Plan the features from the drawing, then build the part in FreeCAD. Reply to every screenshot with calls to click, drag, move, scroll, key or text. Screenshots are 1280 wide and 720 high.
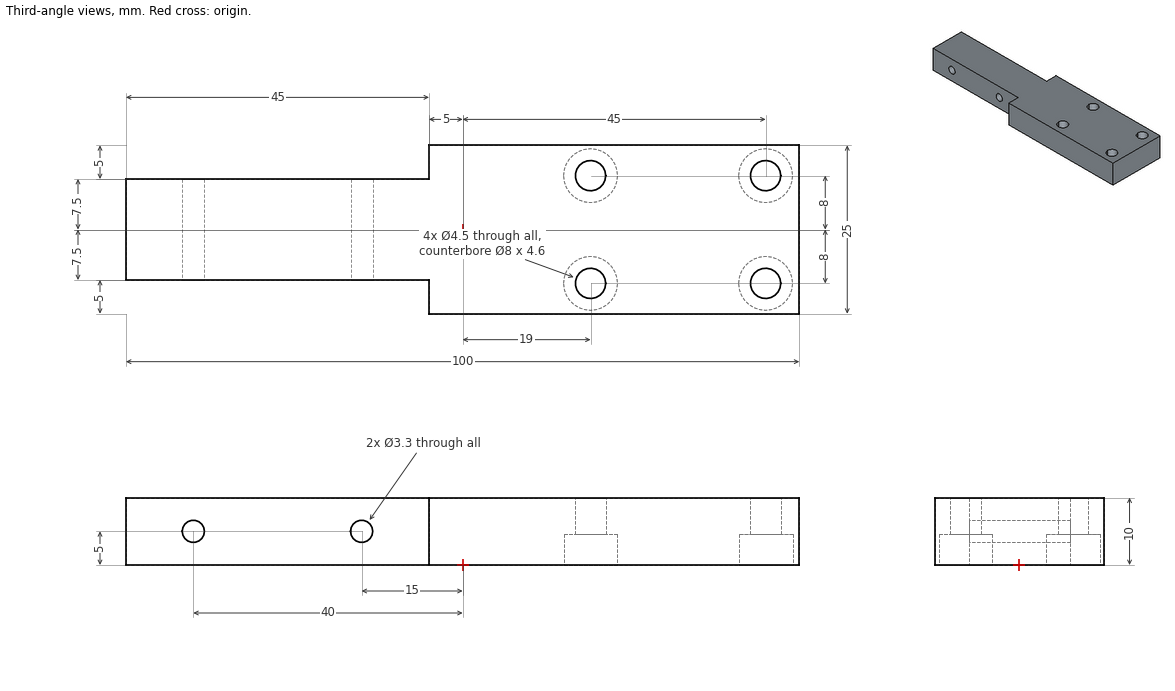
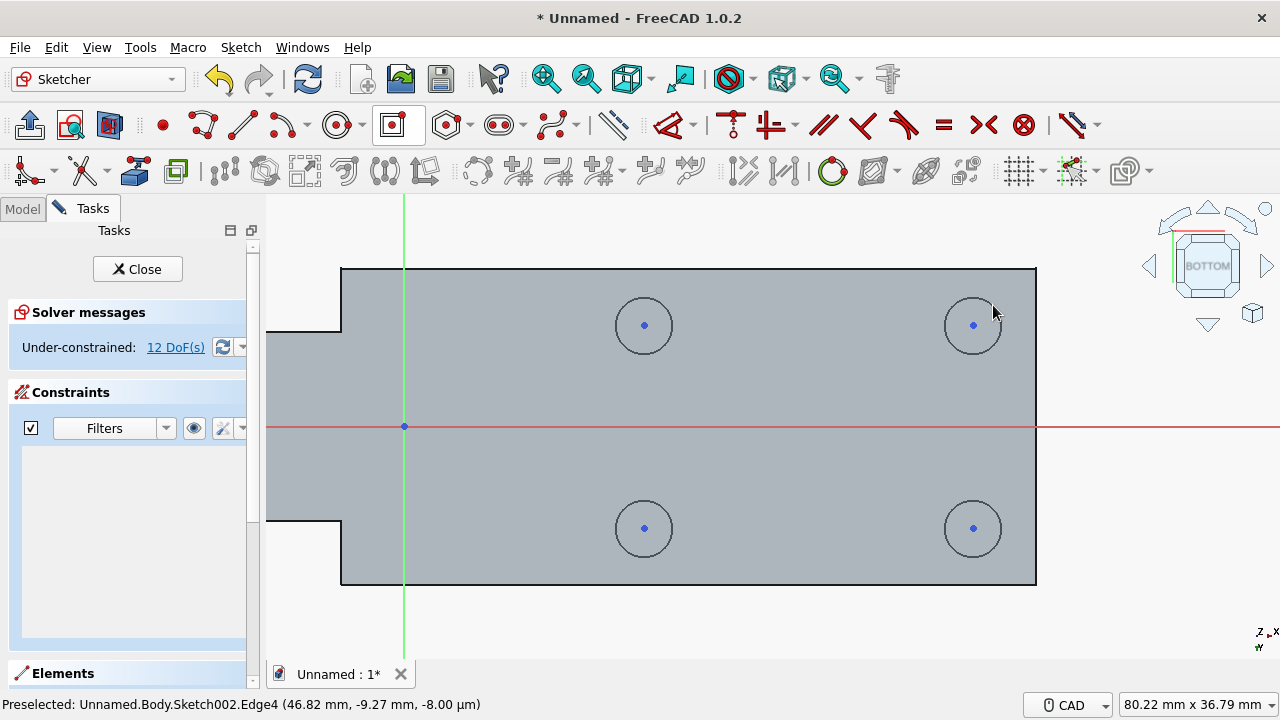
click(664, 306)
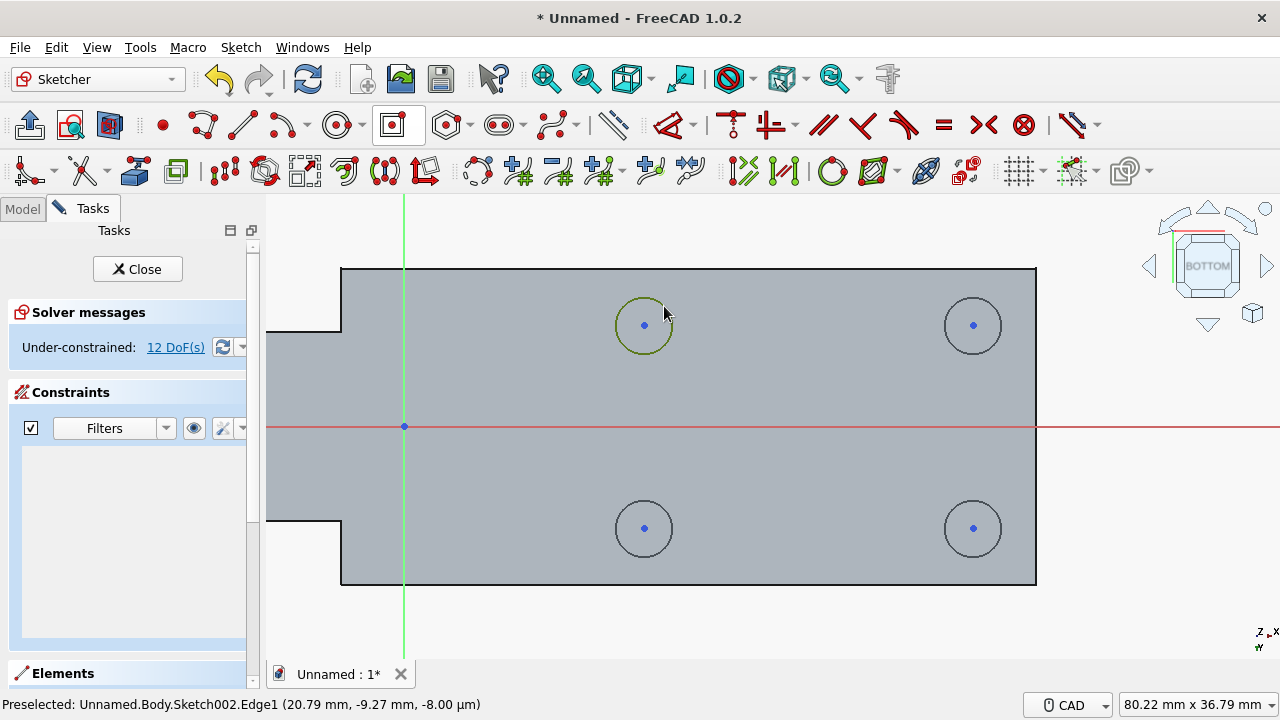
click(664, 509)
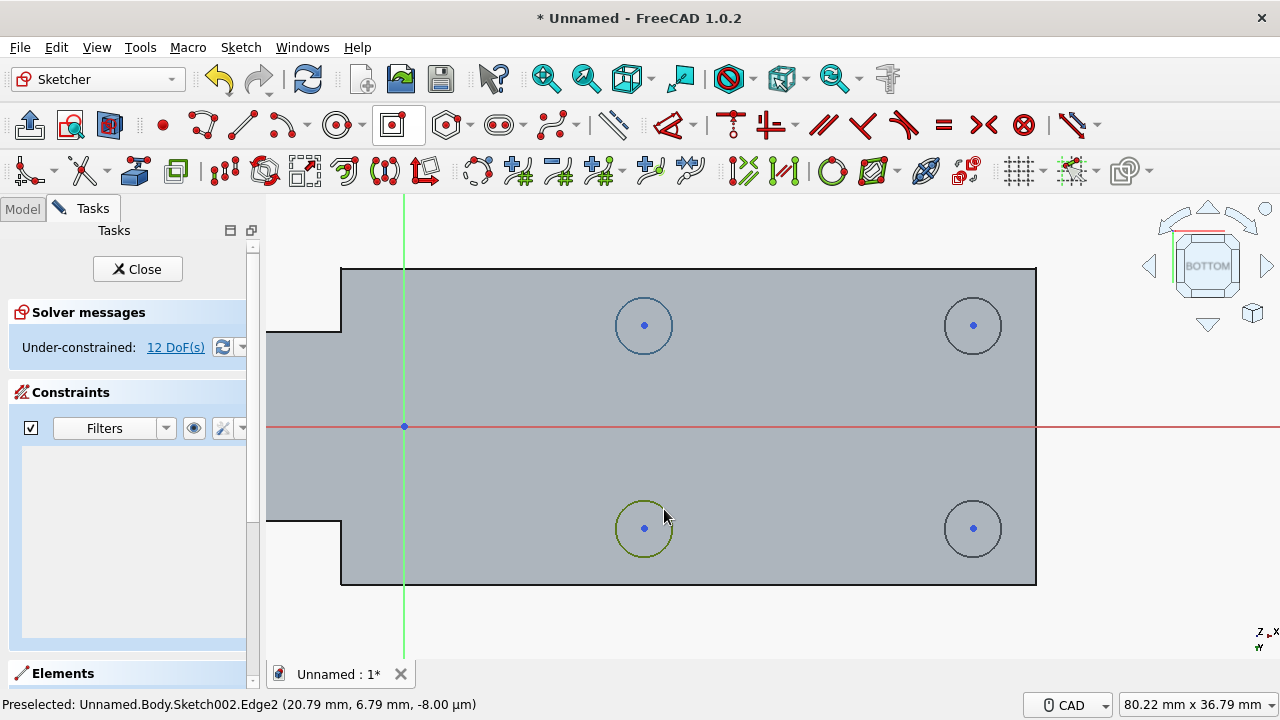
click(993, 509)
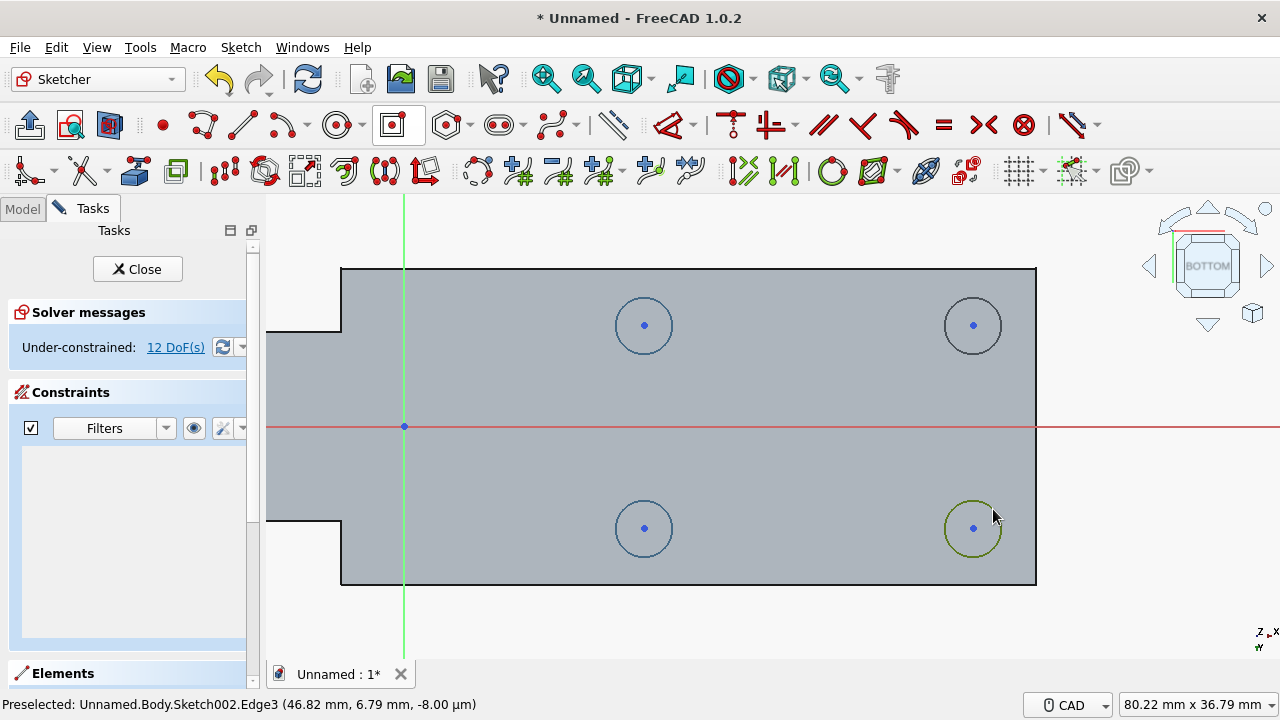
click(993, 306)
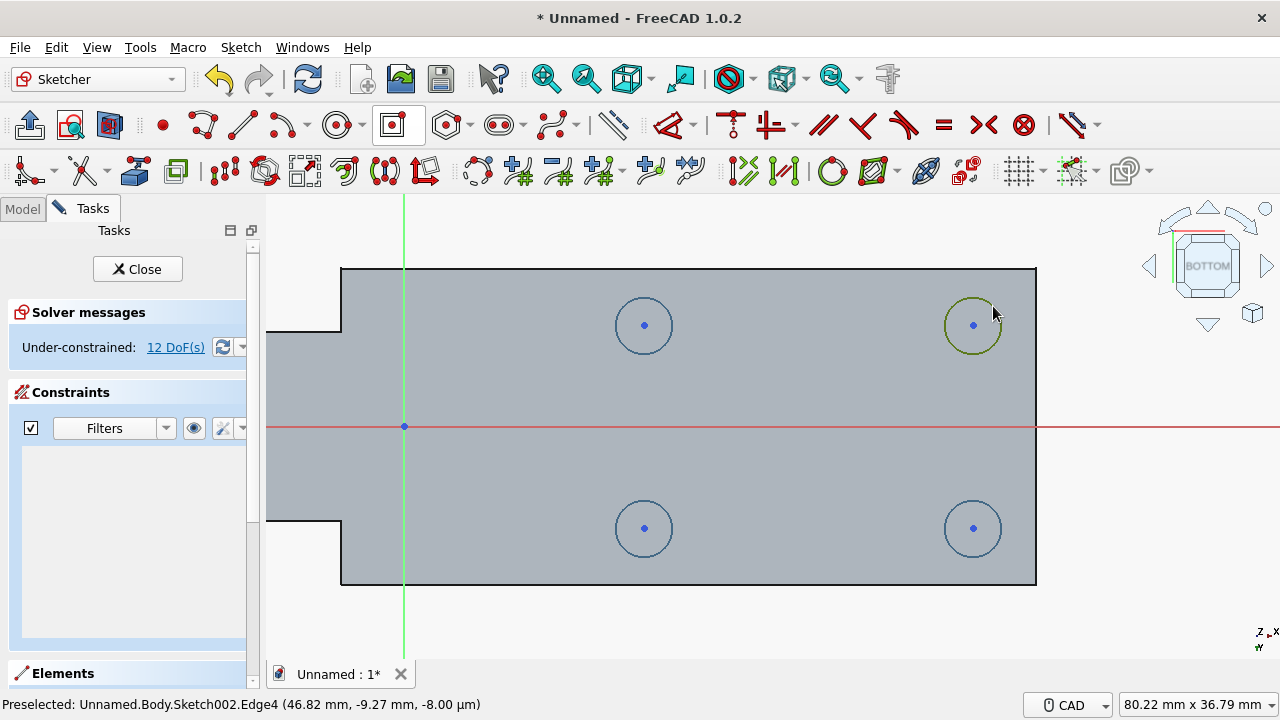
click(944, 126)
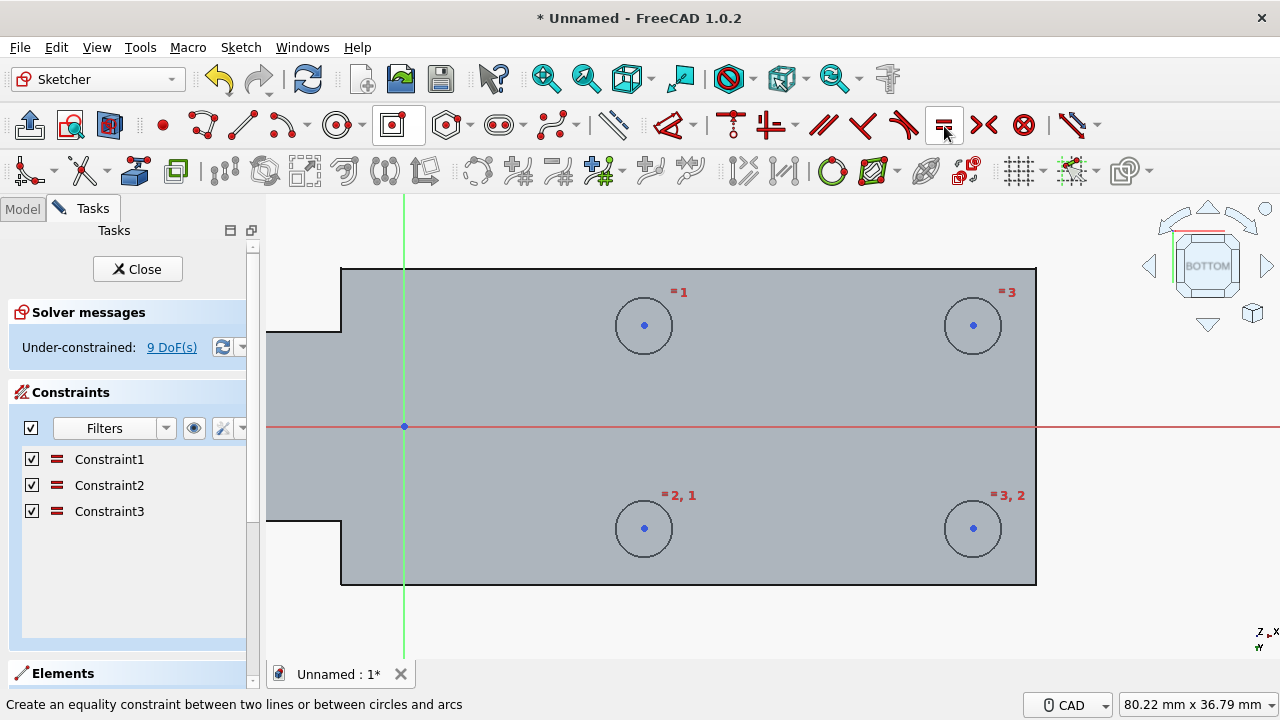
click(644, 326)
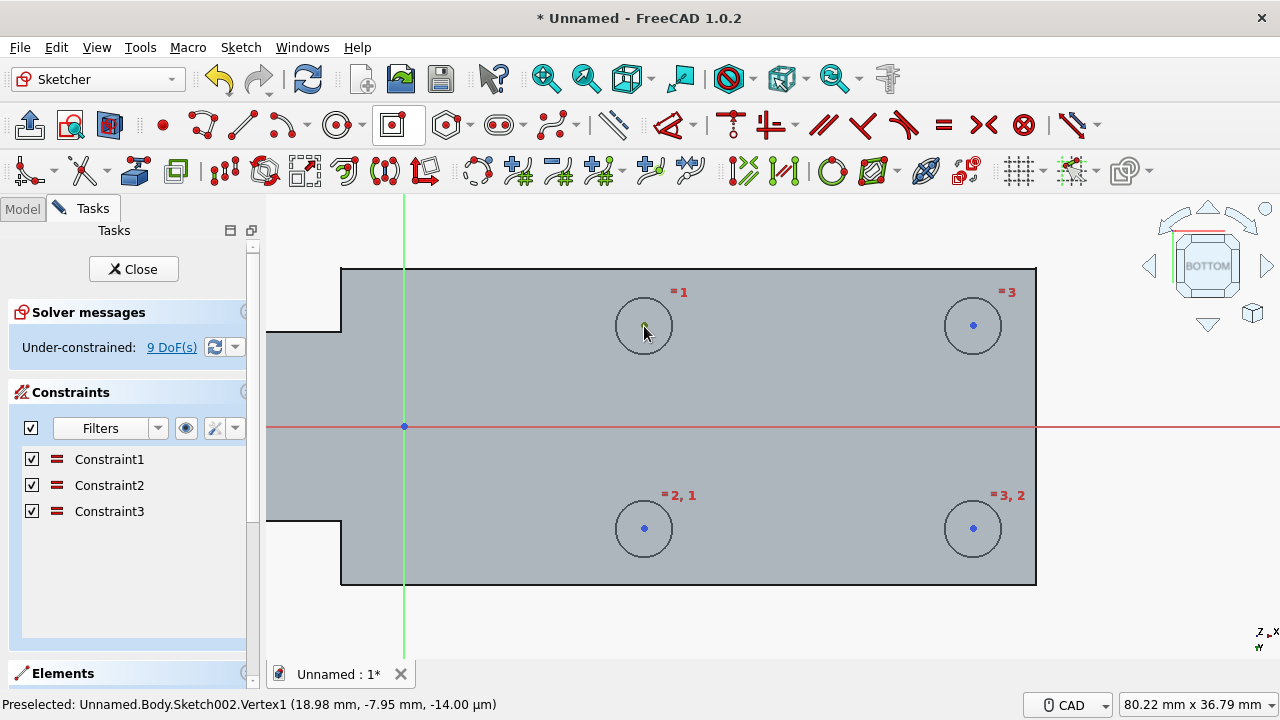
click(644, 529)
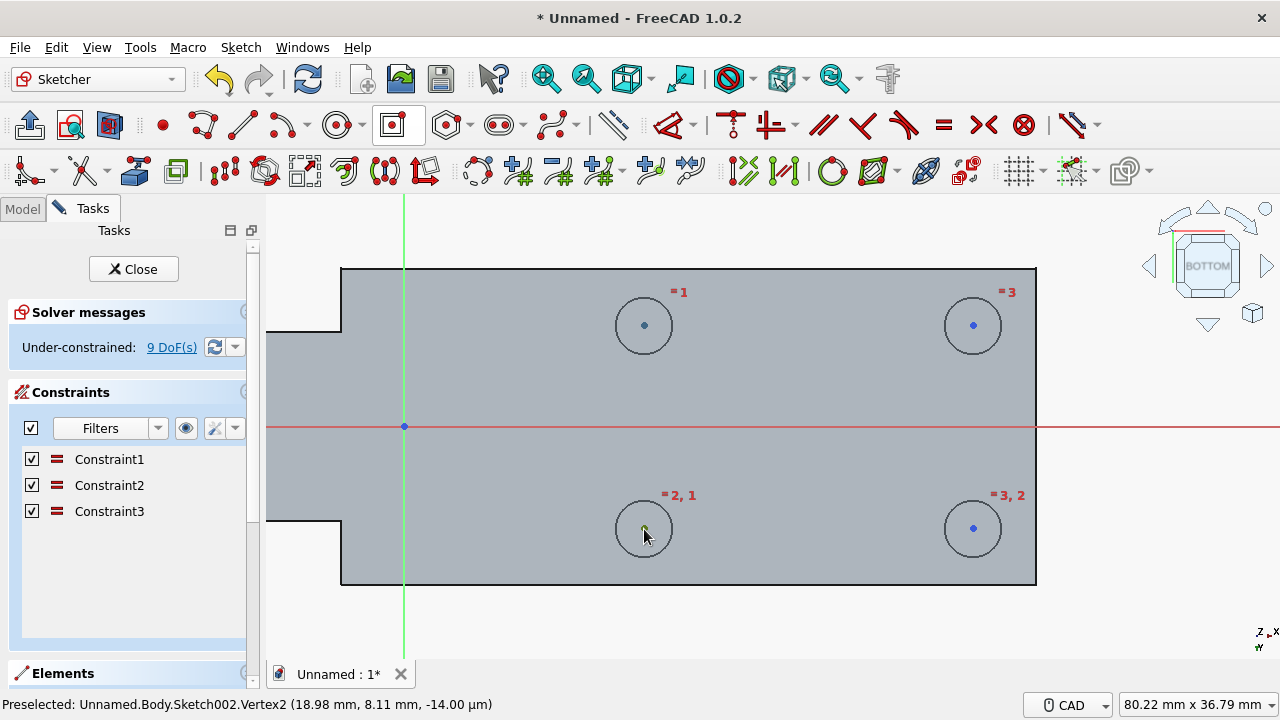
click(798, 126)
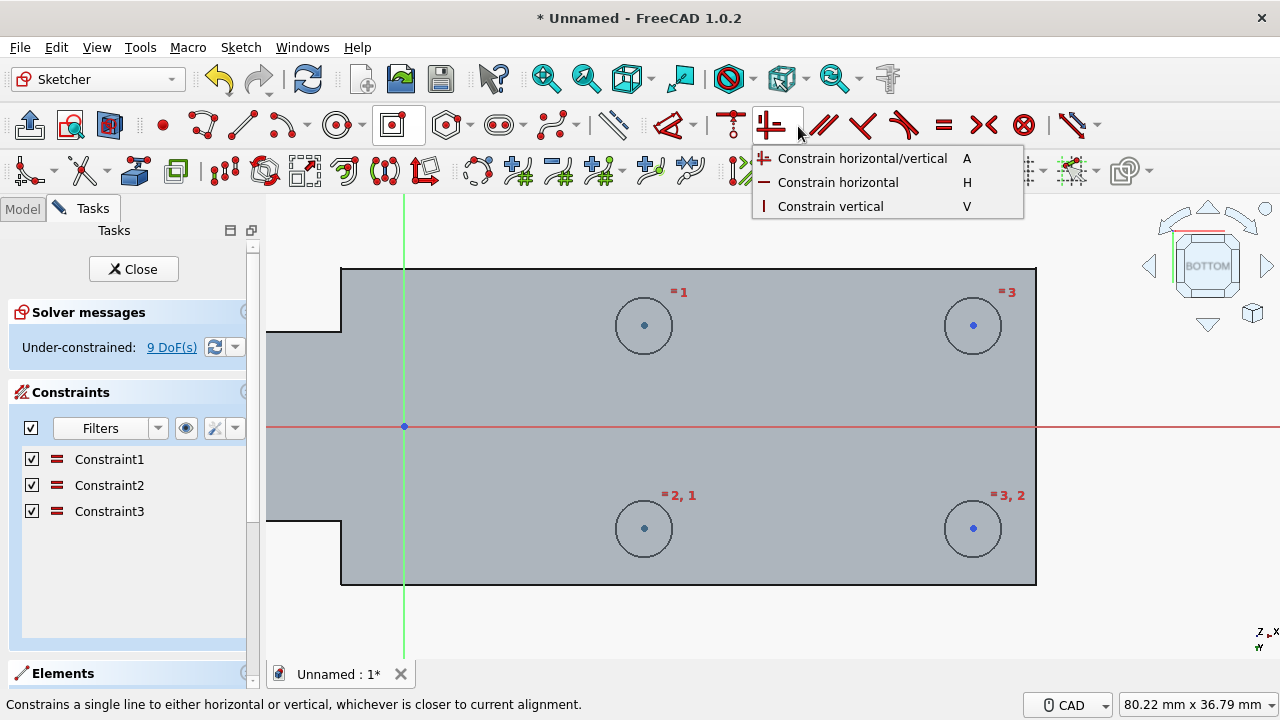
click(888, 206)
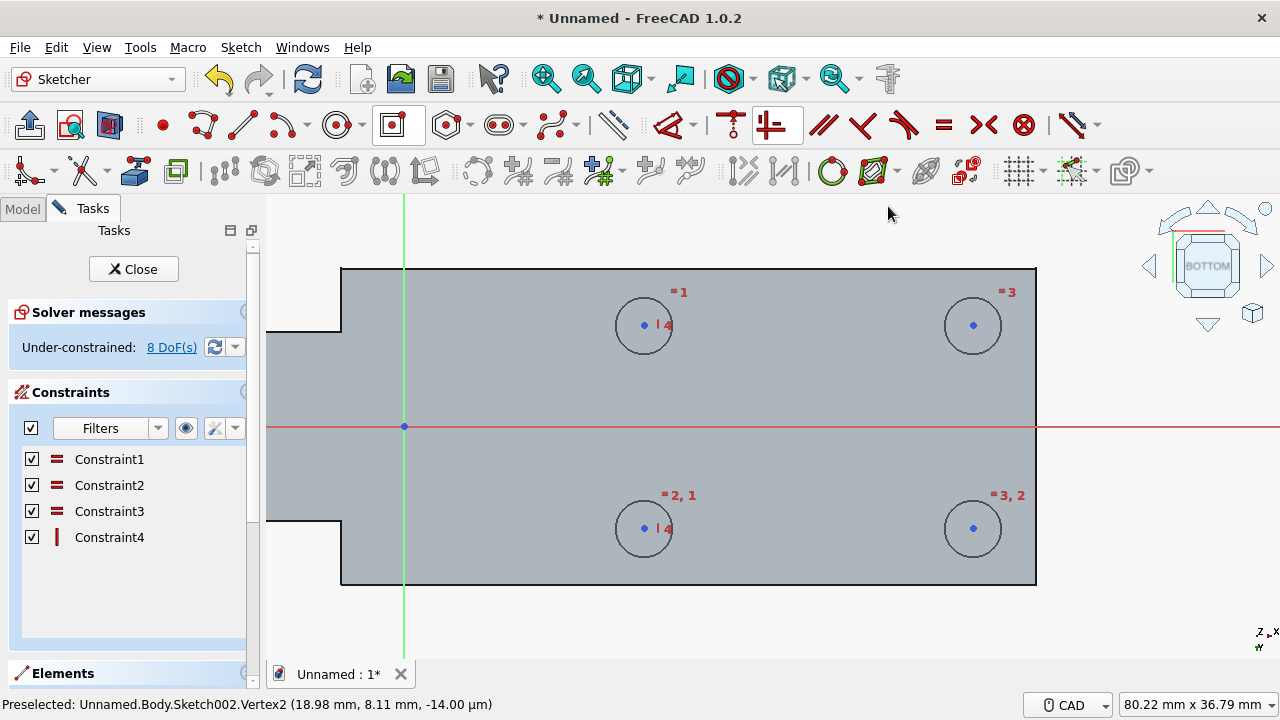
click(644, 529)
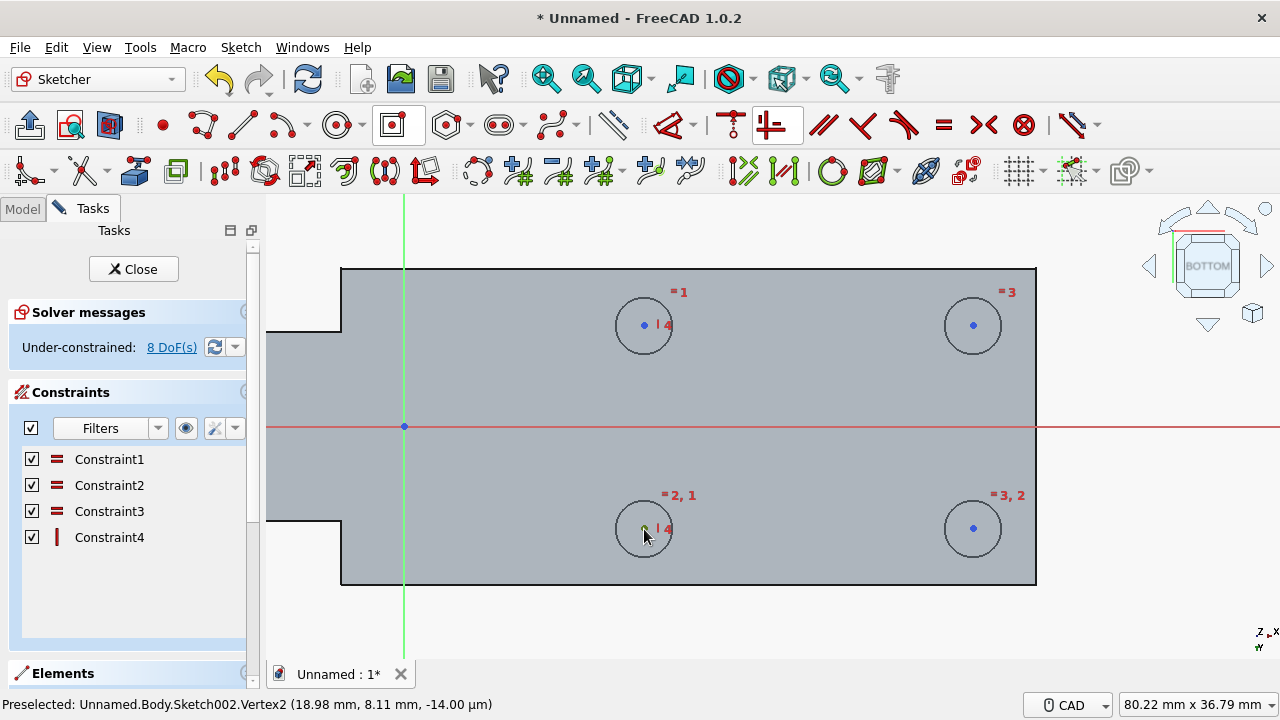
click(973, 529)